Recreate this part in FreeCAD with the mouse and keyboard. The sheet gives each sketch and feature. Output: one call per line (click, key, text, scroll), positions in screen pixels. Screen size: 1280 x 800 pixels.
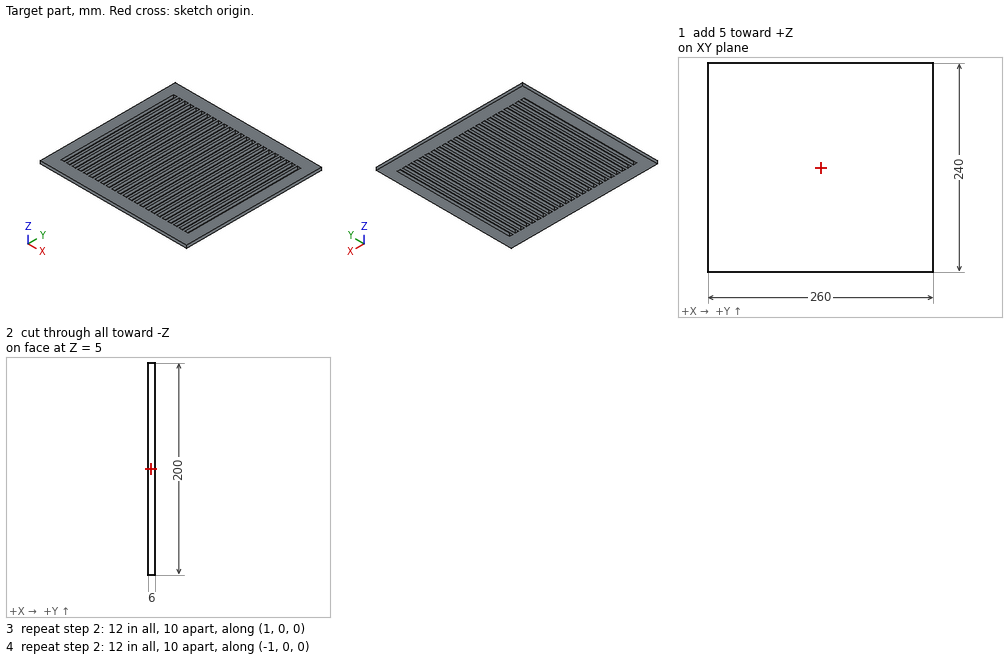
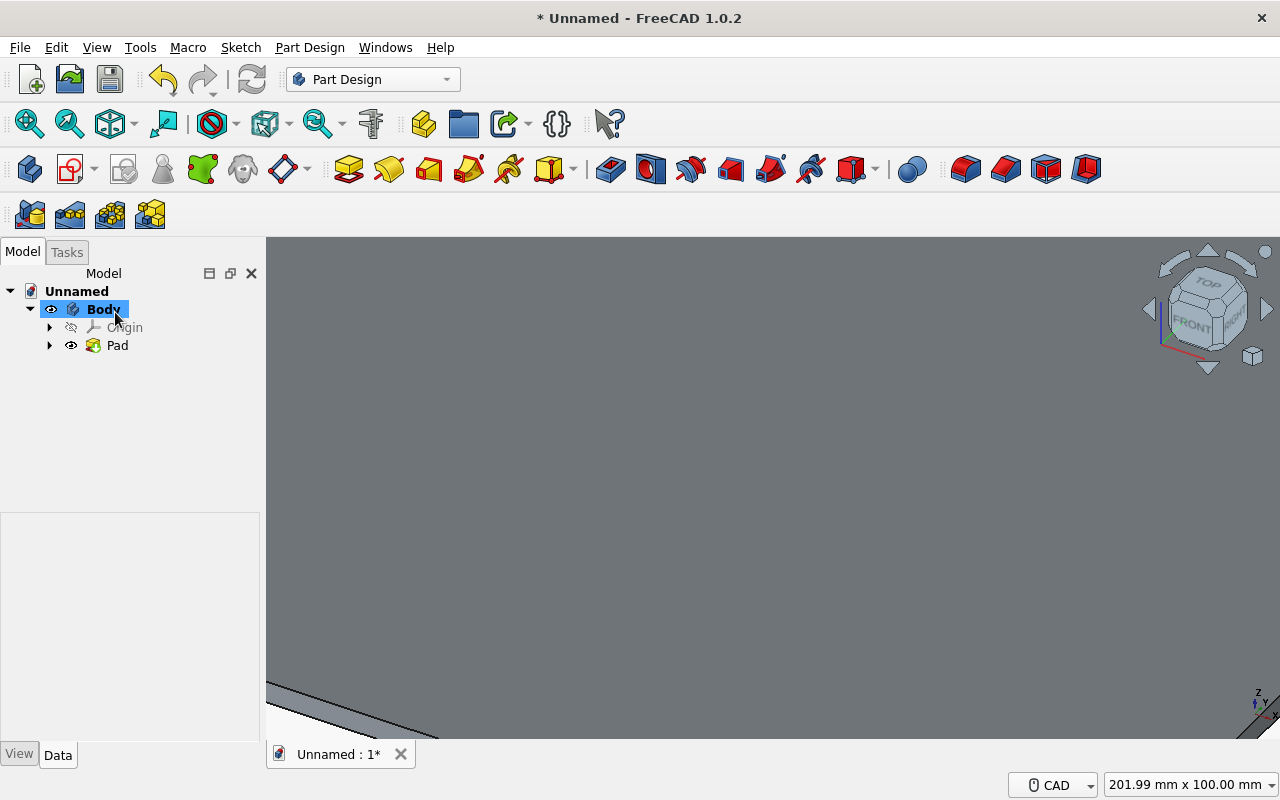
key(v)
key(f)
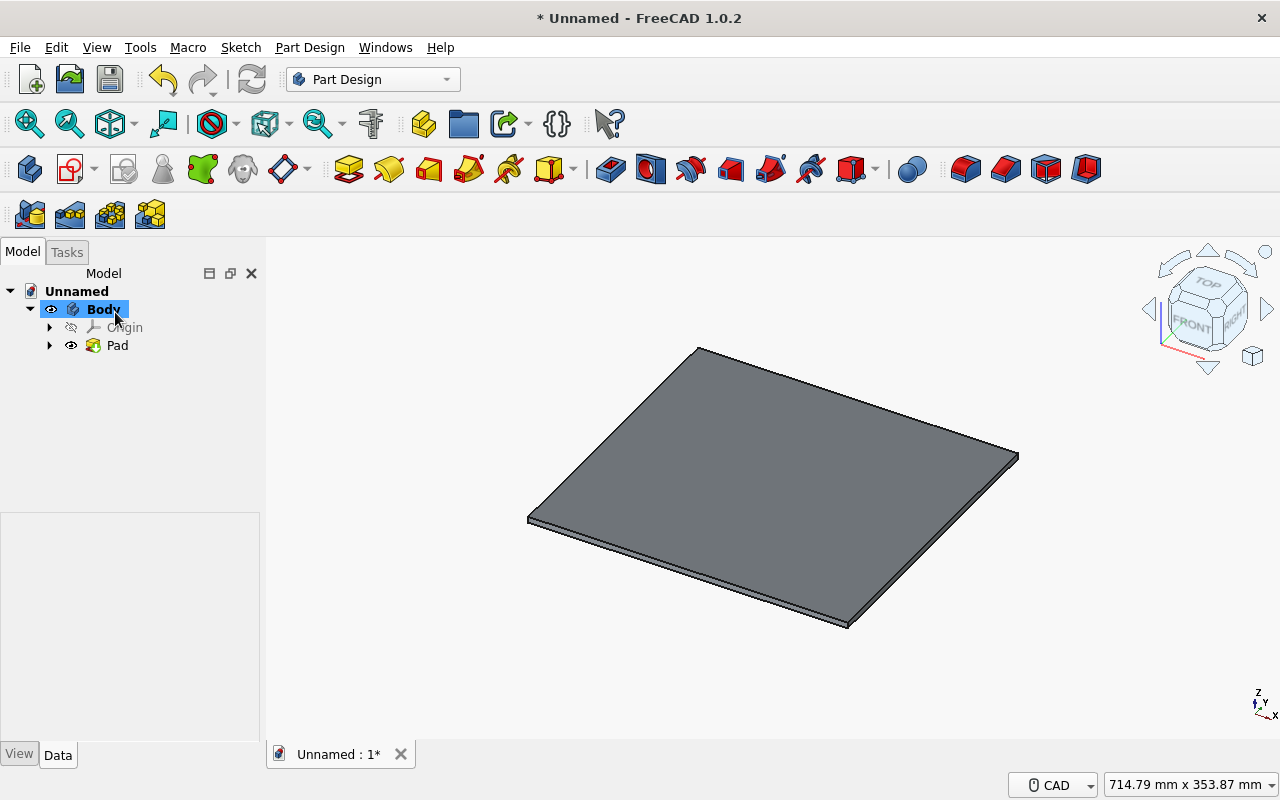
click(773, 484)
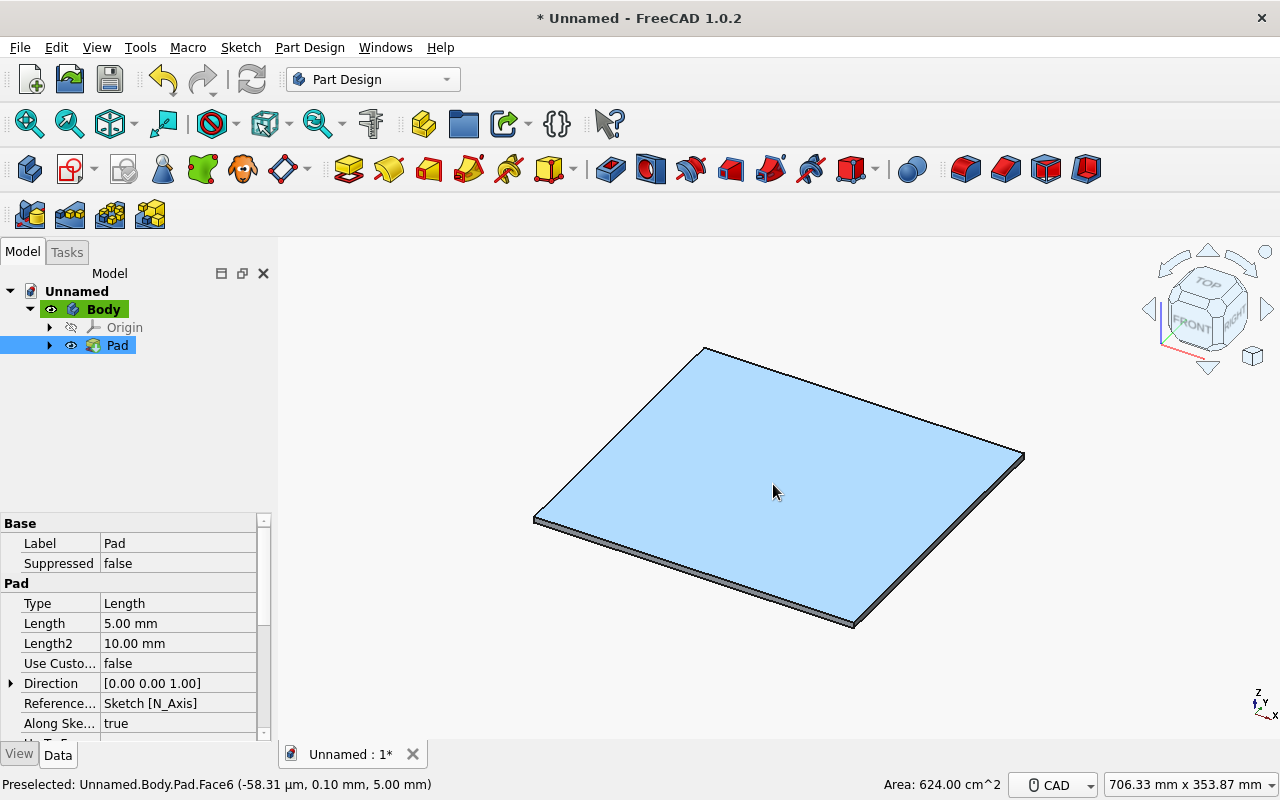
click(70, 170)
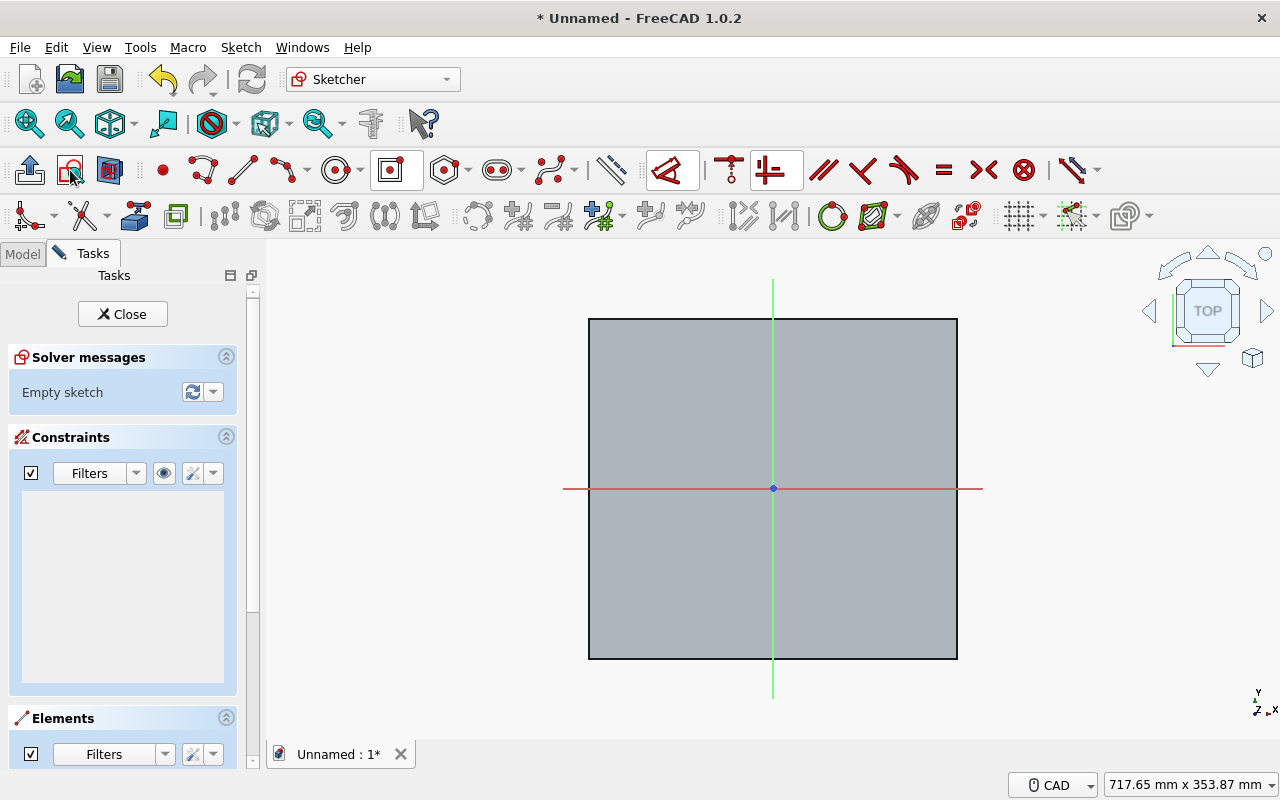
click(390, 170)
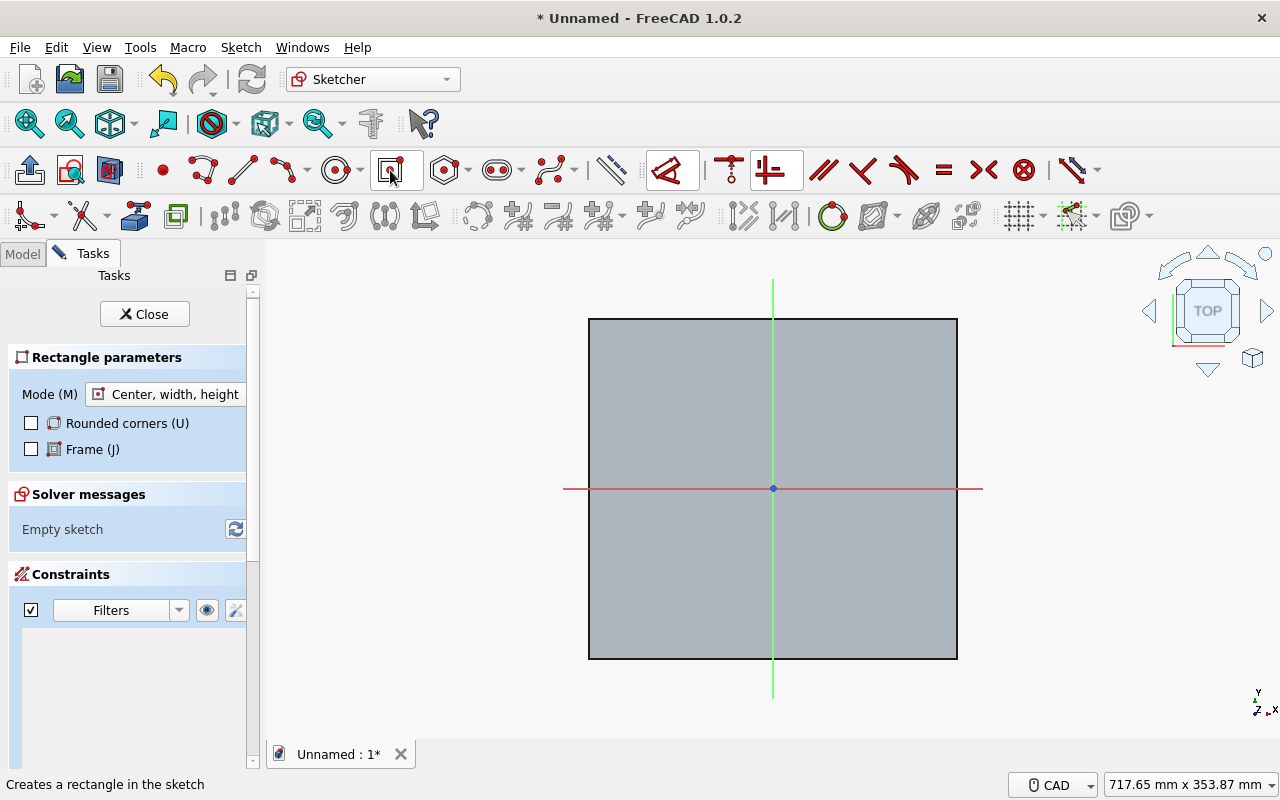
scroll(773, 489, up, 7)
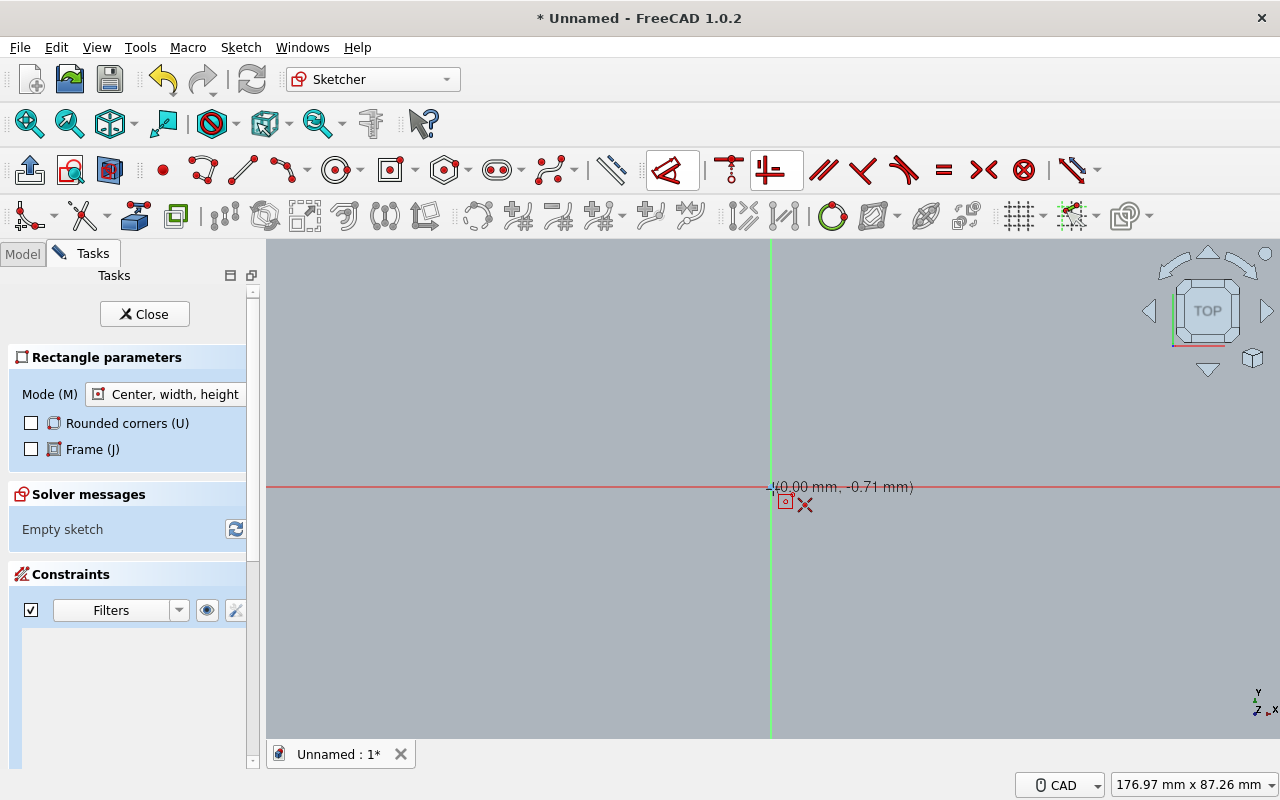
scroll(676, 490, down, 6)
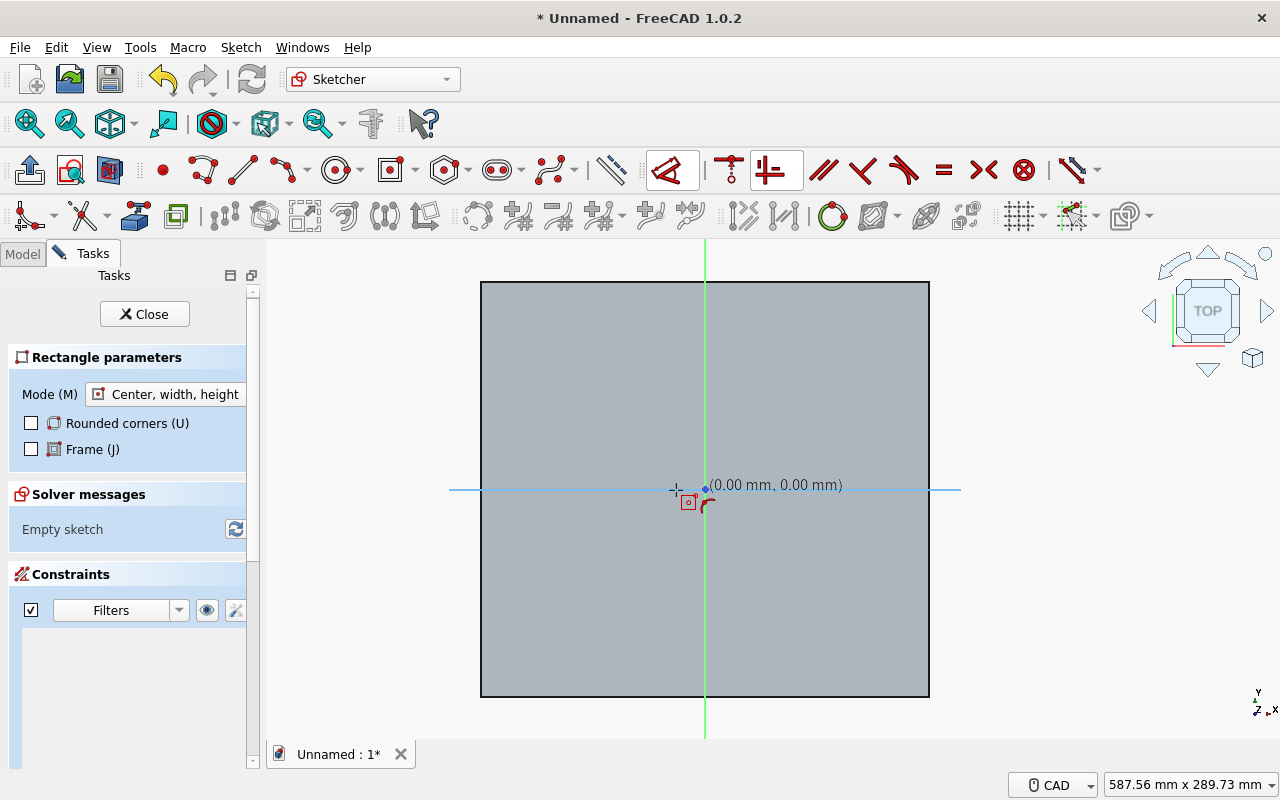
click(705, 490)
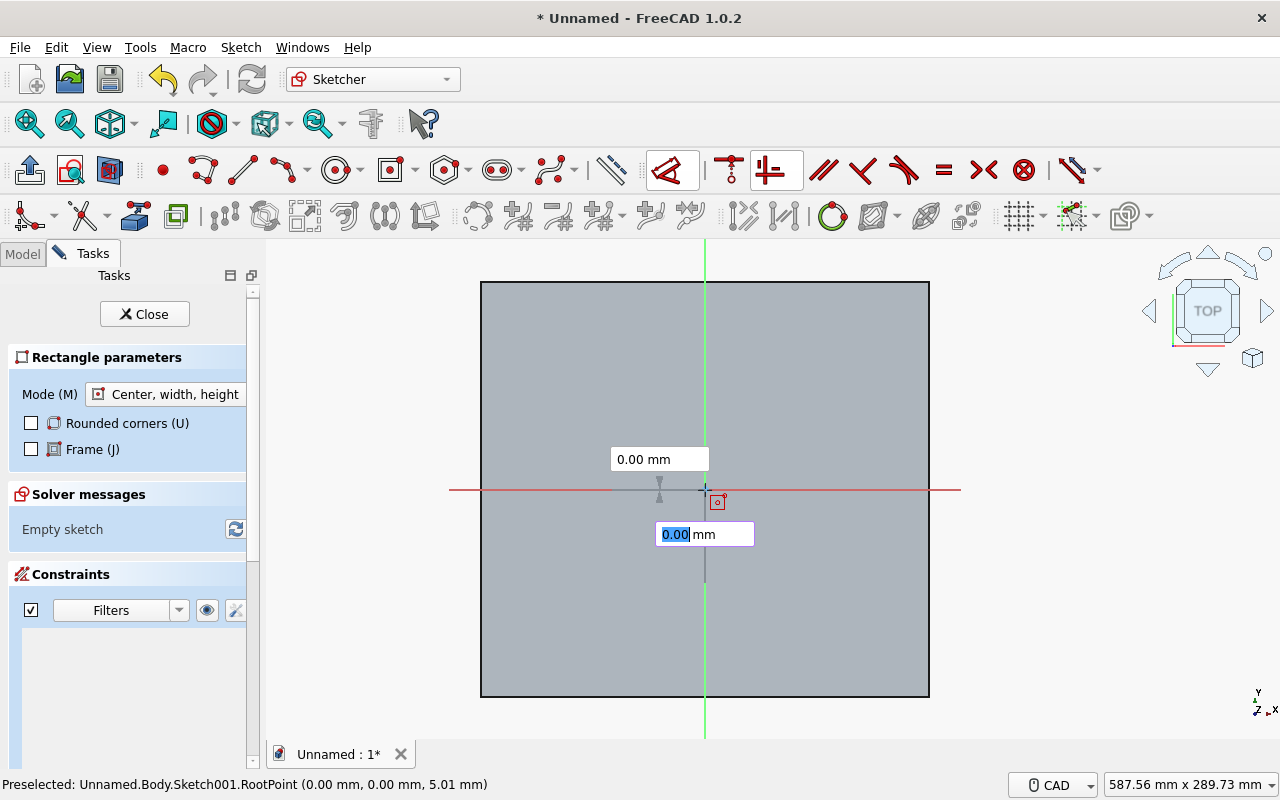
scroll(710, 317, up, 6)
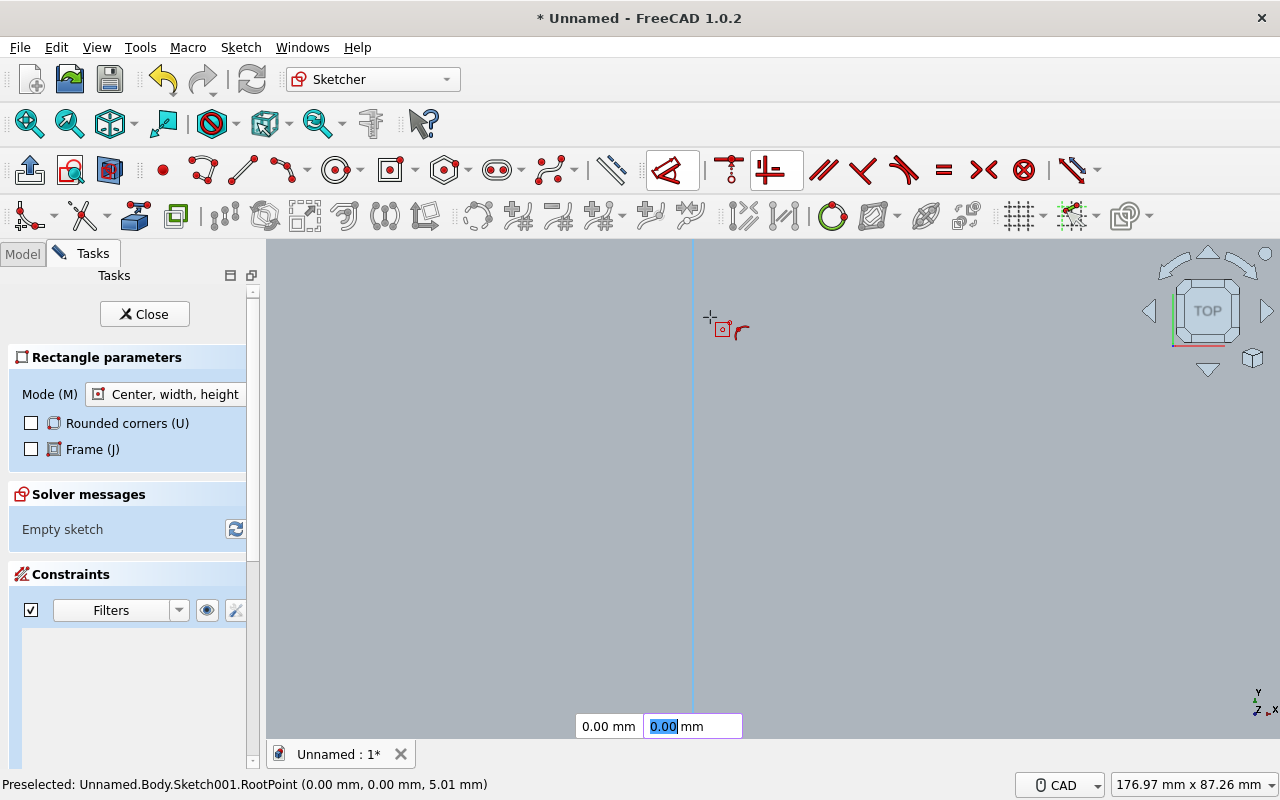
click(710, 317)
key(Escape)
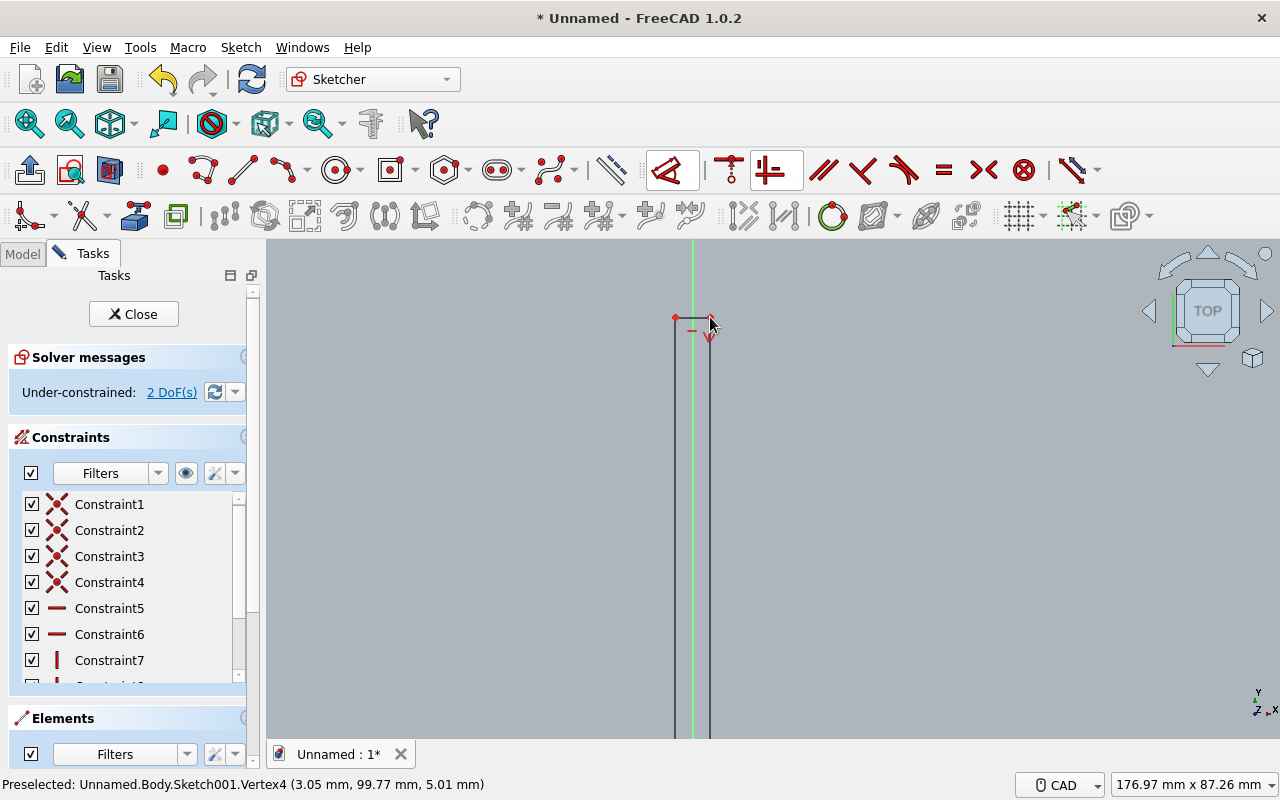
scroll(710, 316, down, 6)